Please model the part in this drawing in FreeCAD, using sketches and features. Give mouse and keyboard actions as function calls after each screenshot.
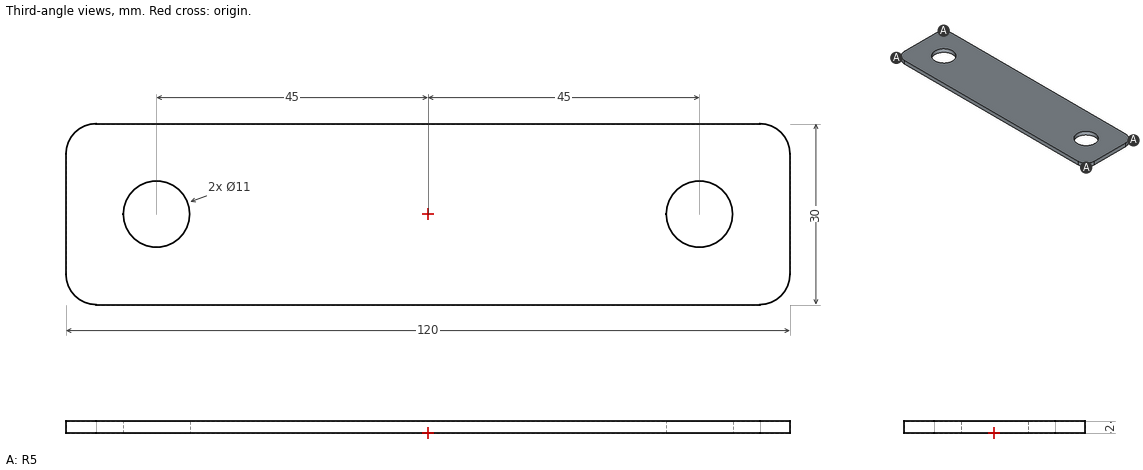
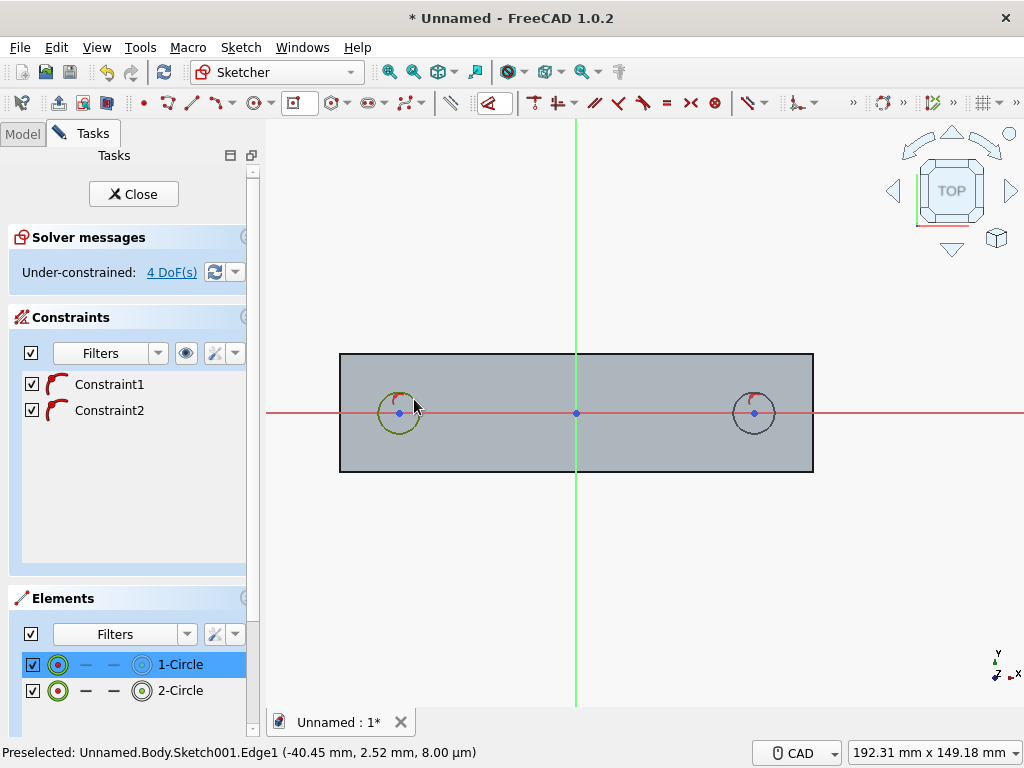
click(769, 399)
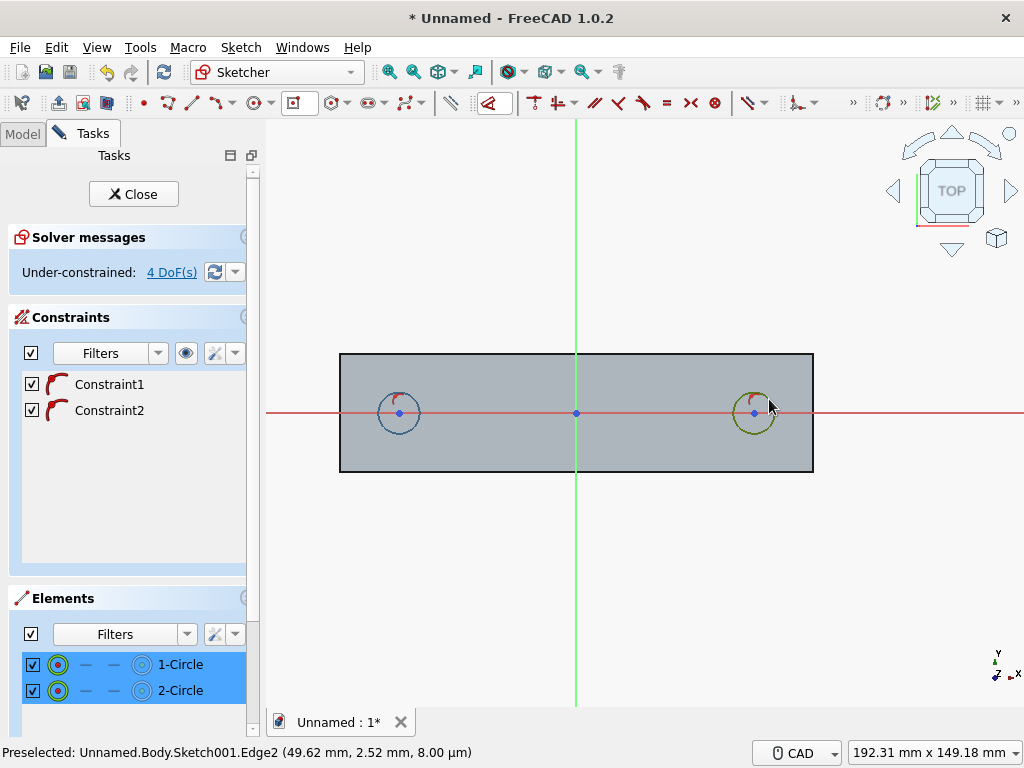
click(668, 104)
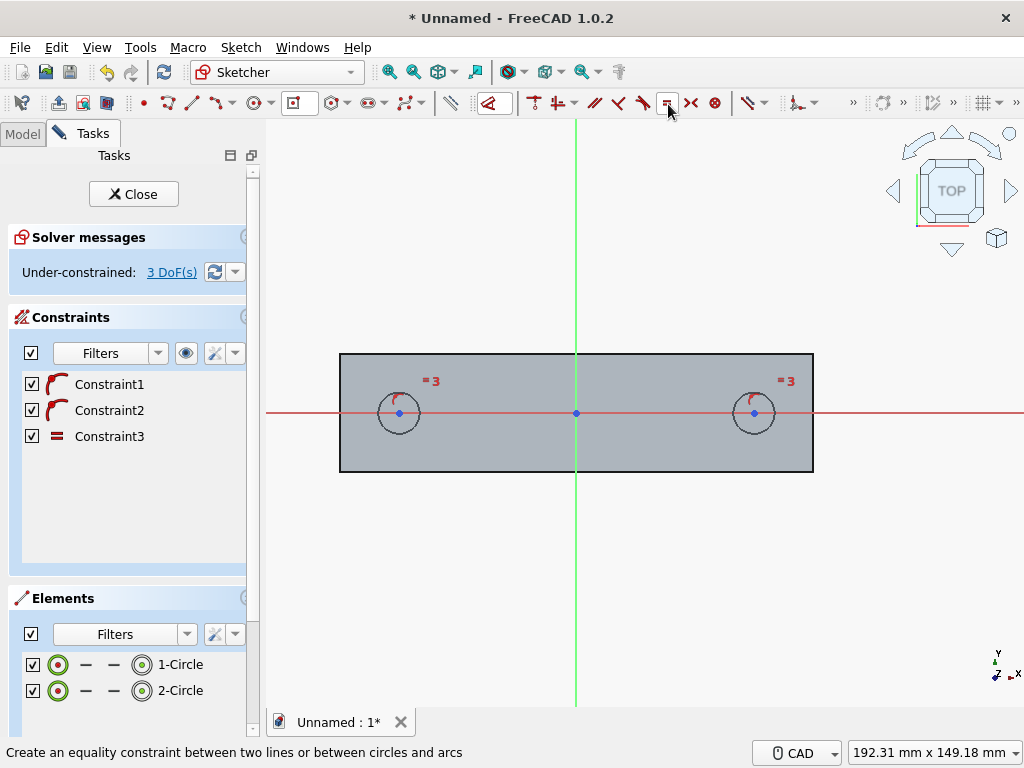
key(d)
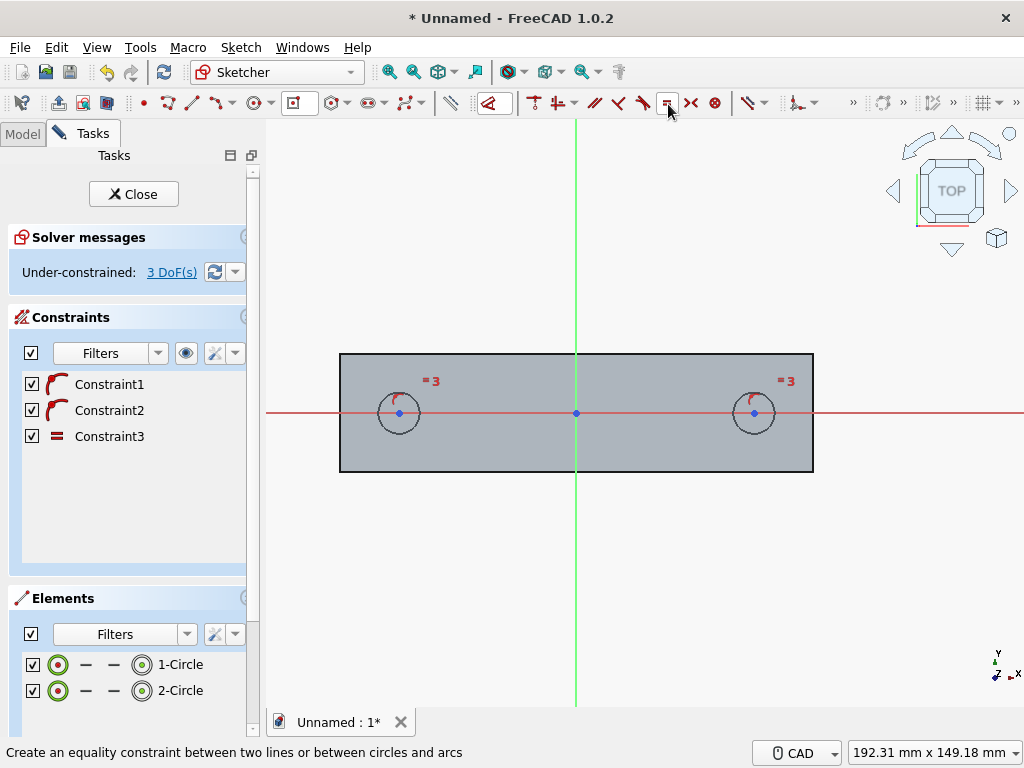
click(414, 399)
click(437, 377)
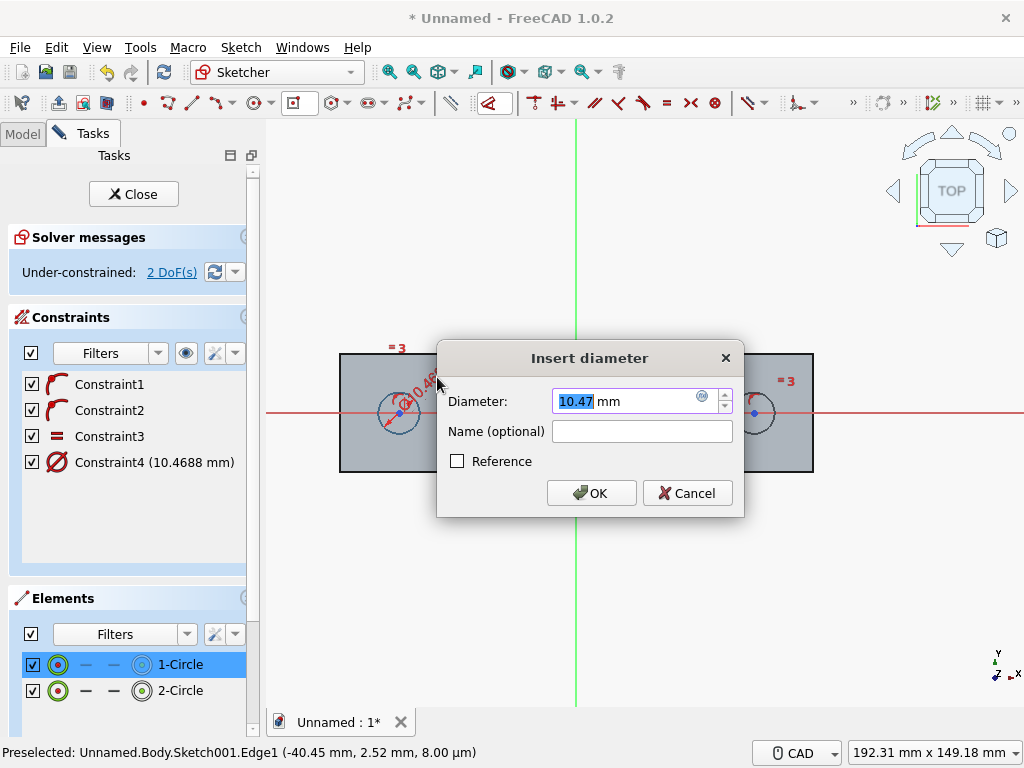
text(11)
key(Return)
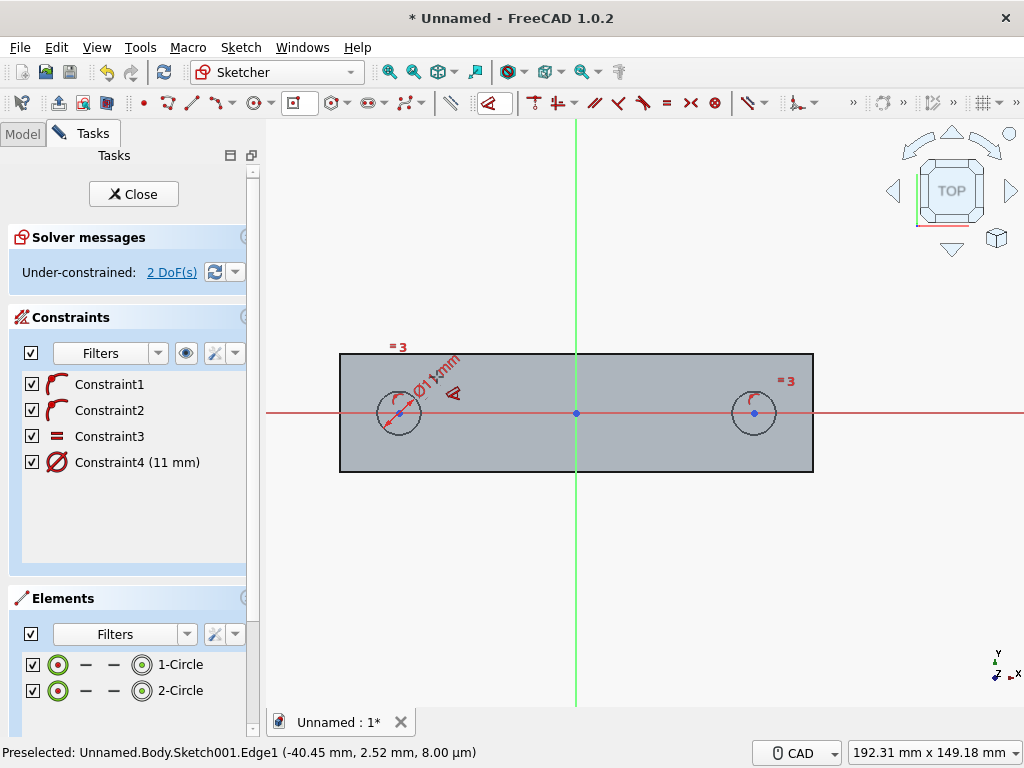
click(399, 413)
click(488, 447)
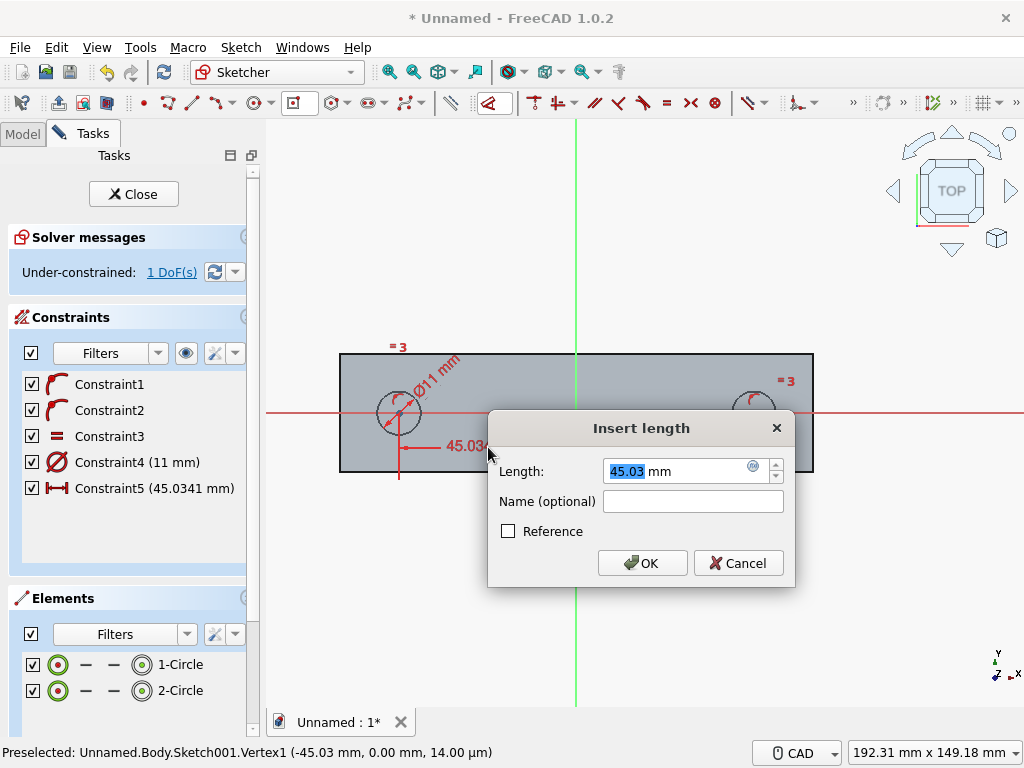
text(45)
key(Return)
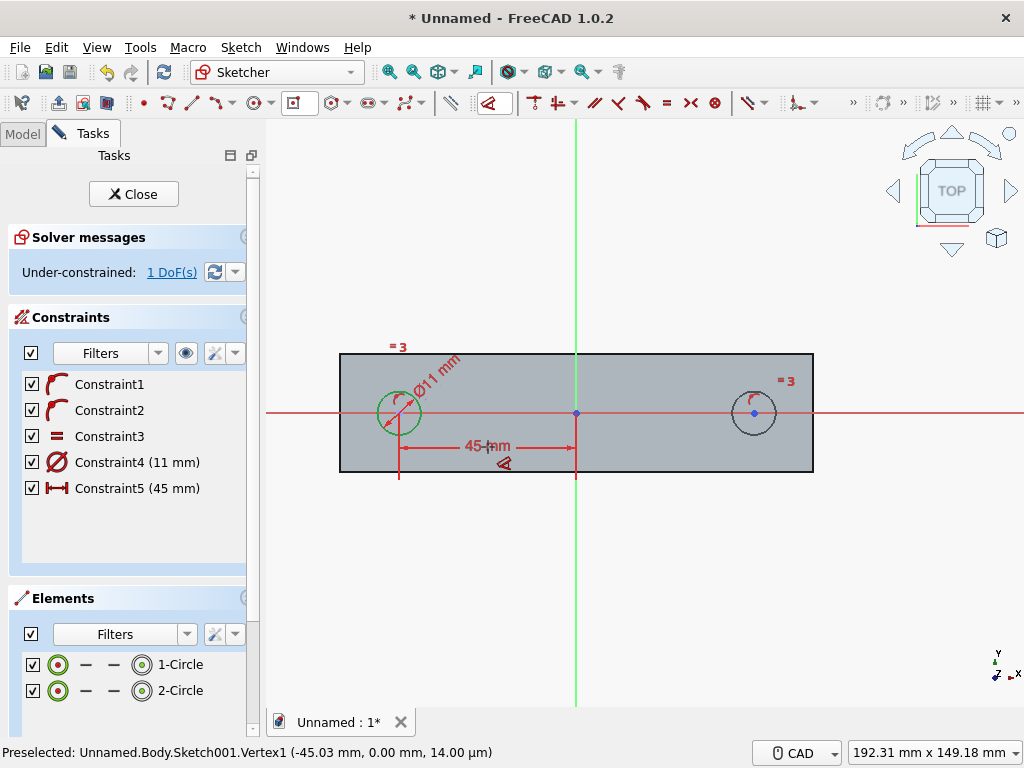
click(754, 413)
click(665, 447)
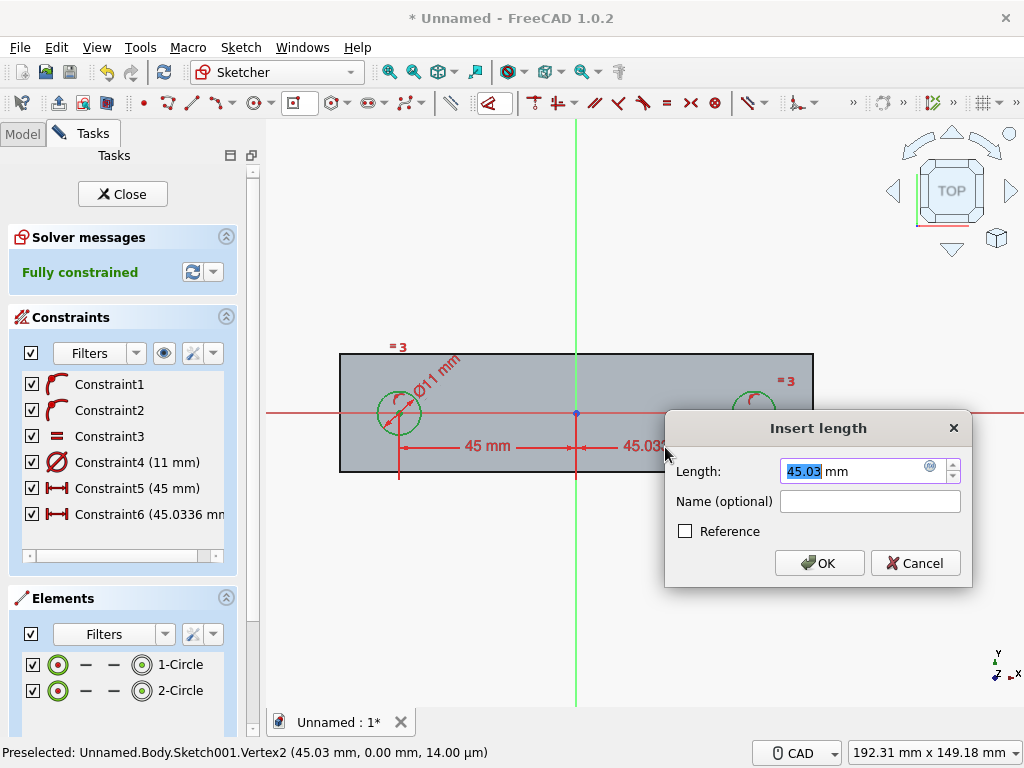
text(45)
key(Return)
key(Escape)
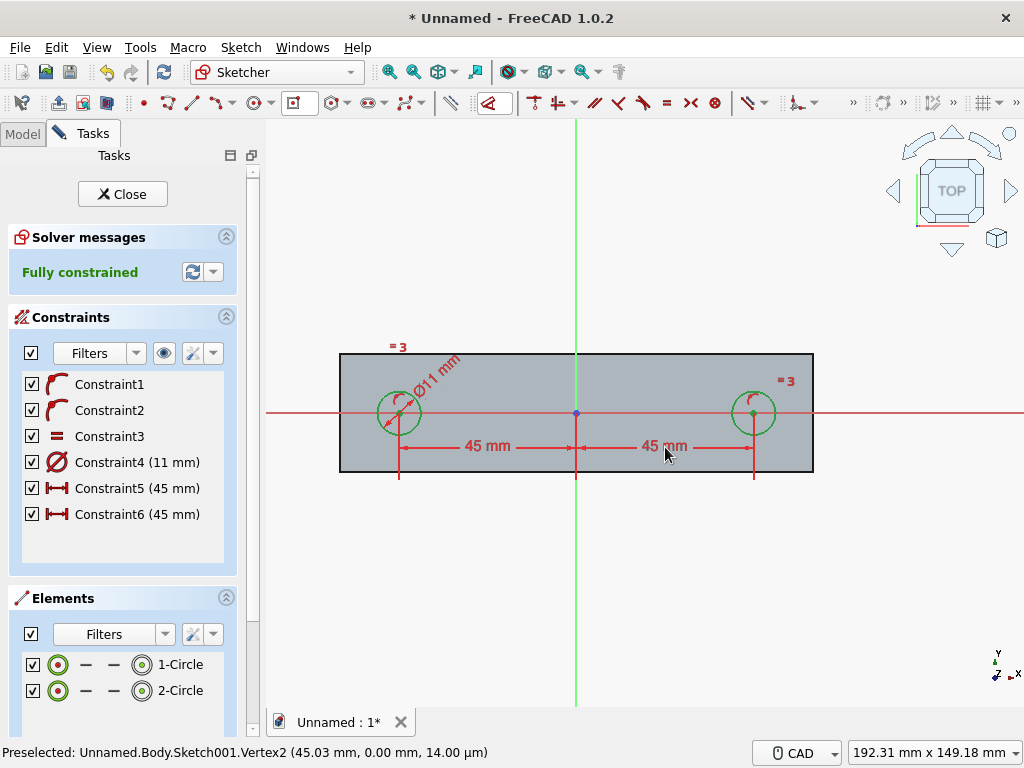
click(123, 194)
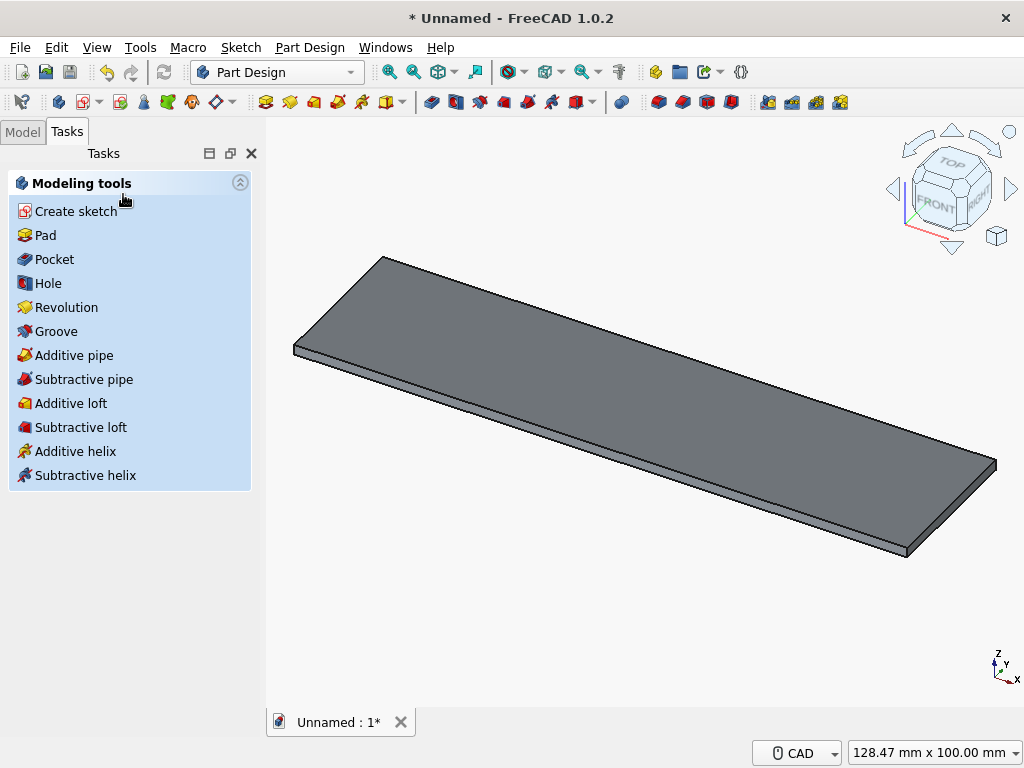
click(432, 102)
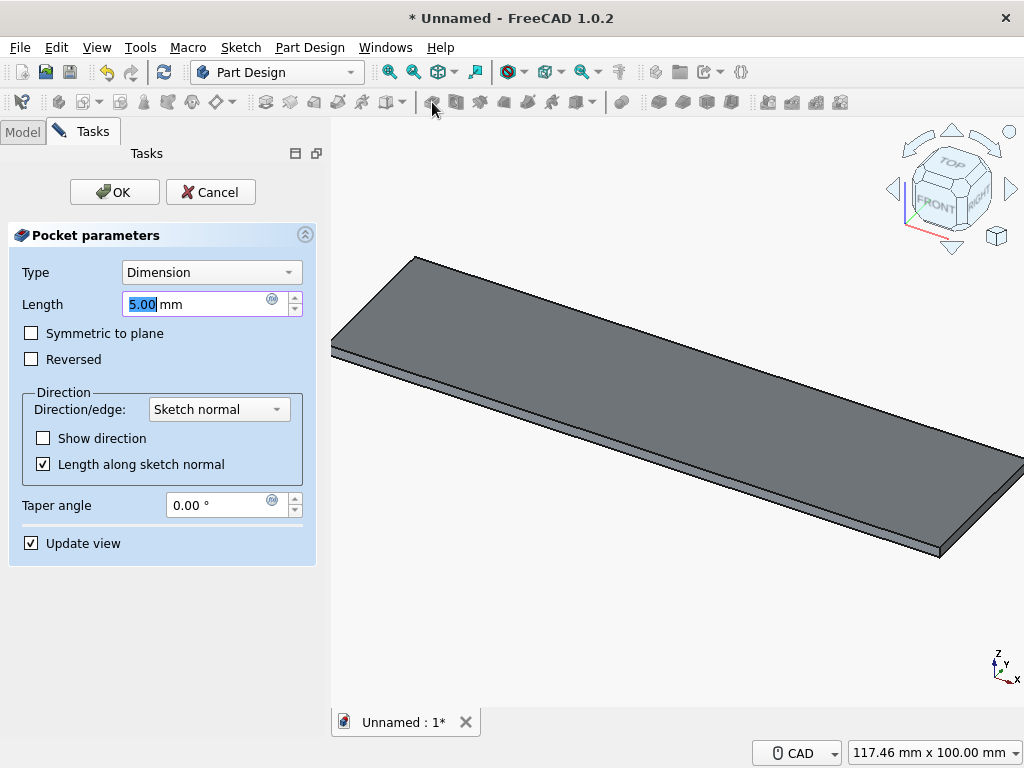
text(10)
key(Tab)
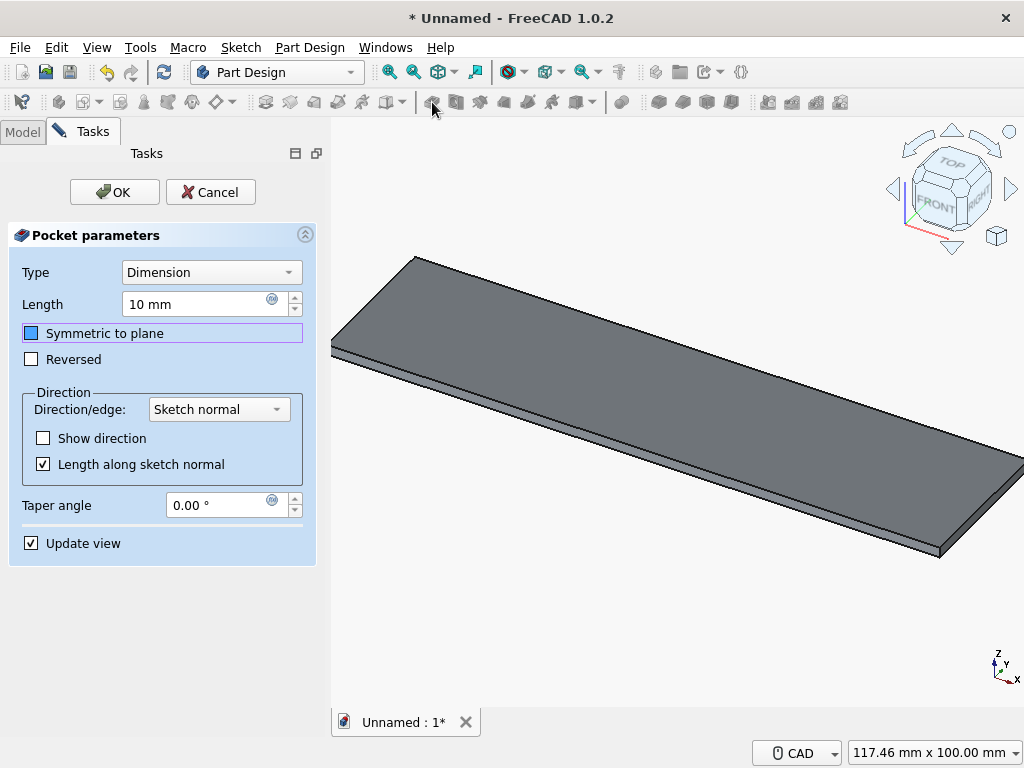
click(30, 359)